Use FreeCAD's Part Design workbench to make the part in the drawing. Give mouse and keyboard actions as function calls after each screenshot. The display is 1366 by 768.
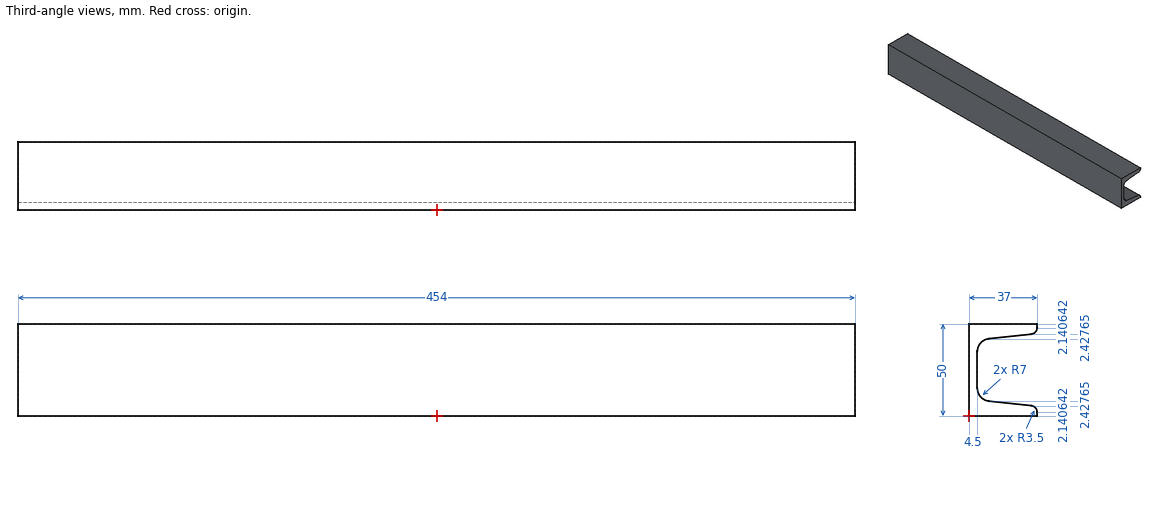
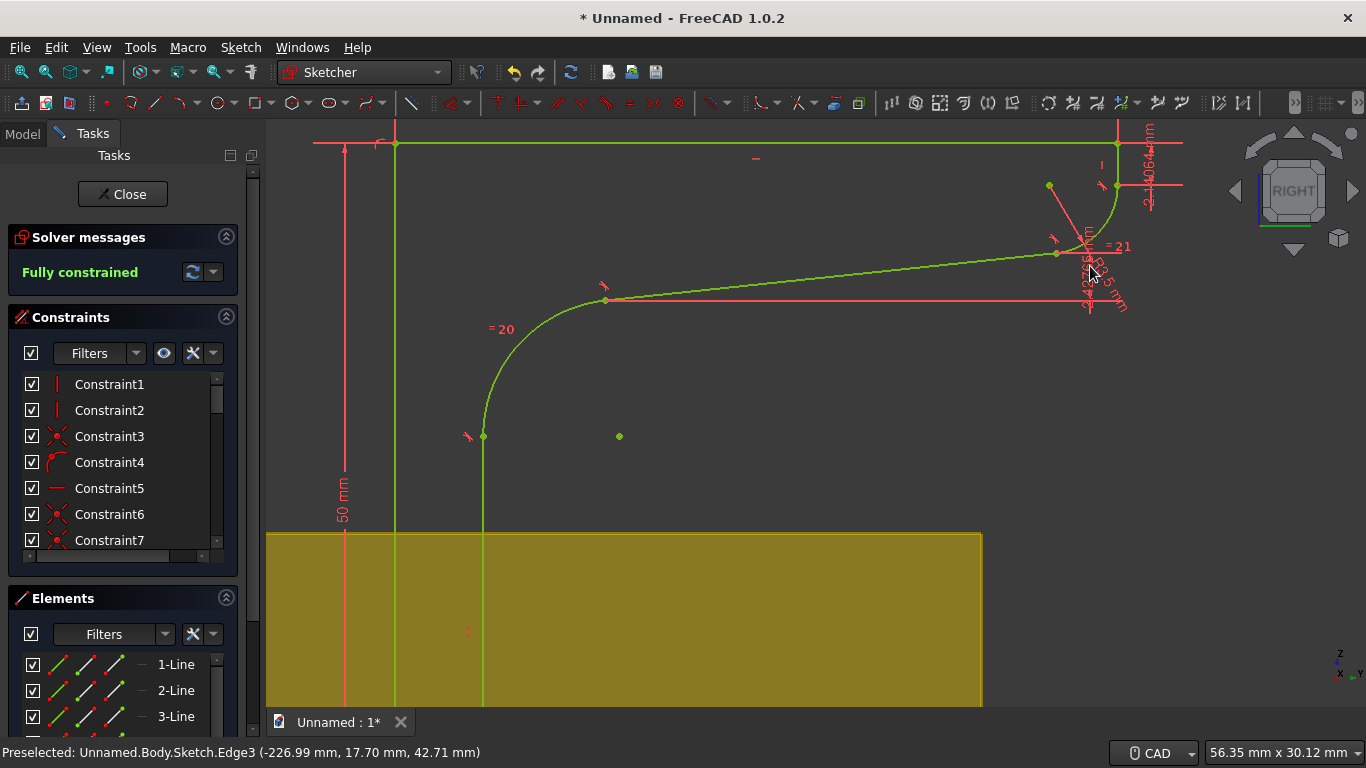
click(123, 194)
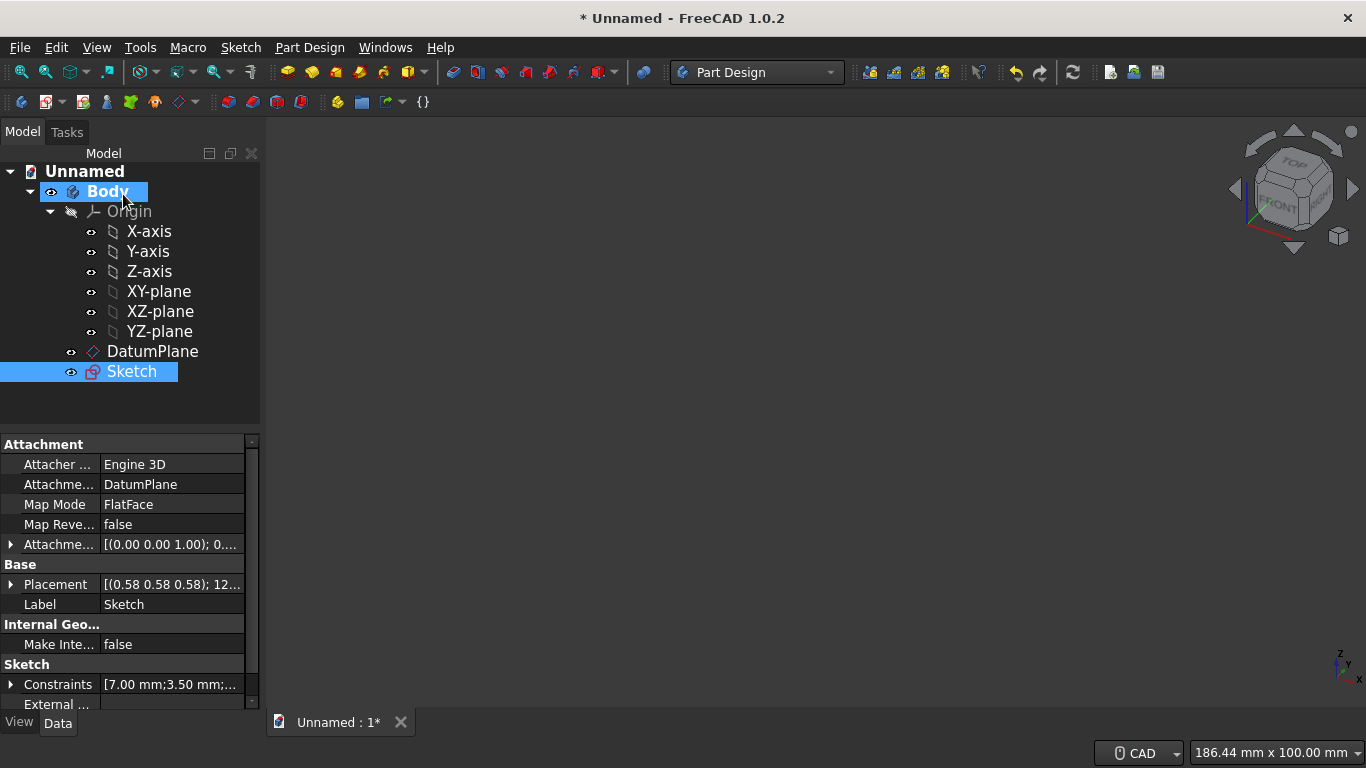
click(288, 72)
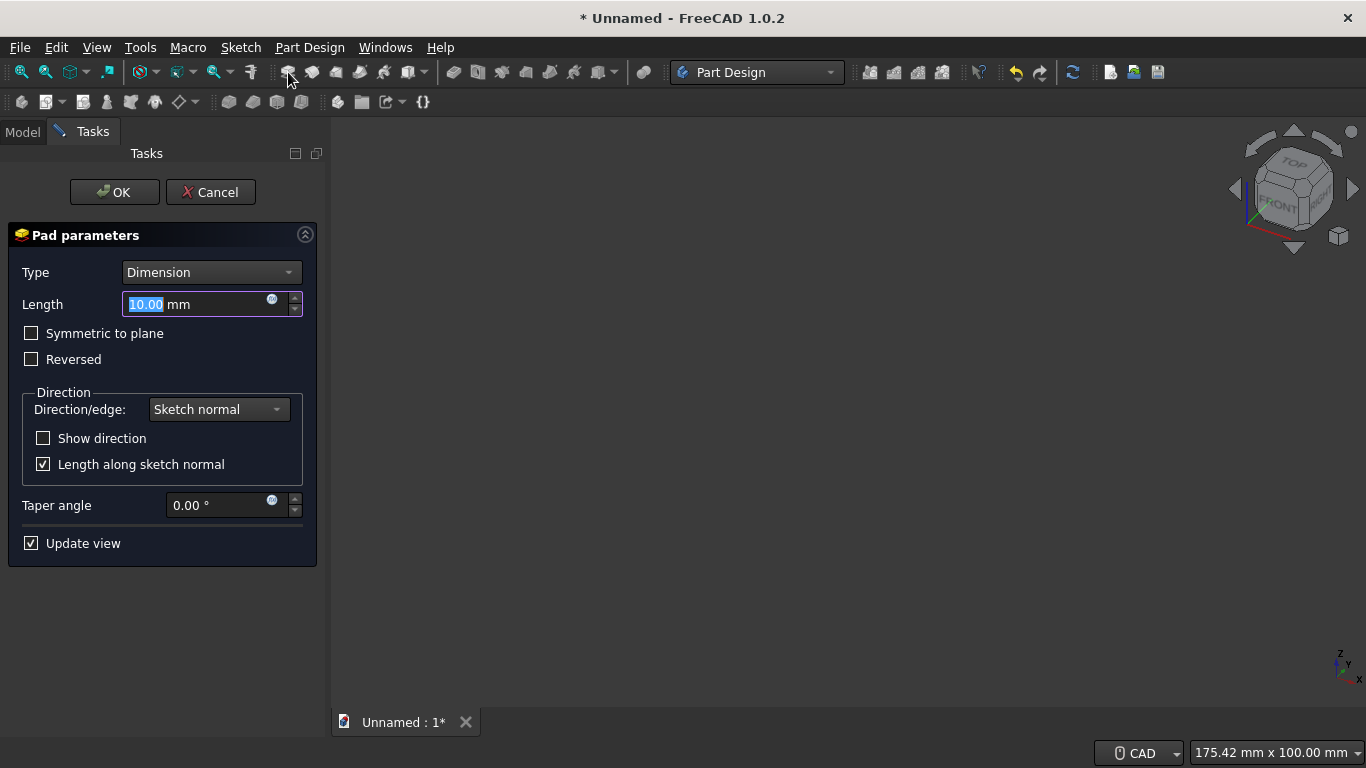
text(454)
key(Tab)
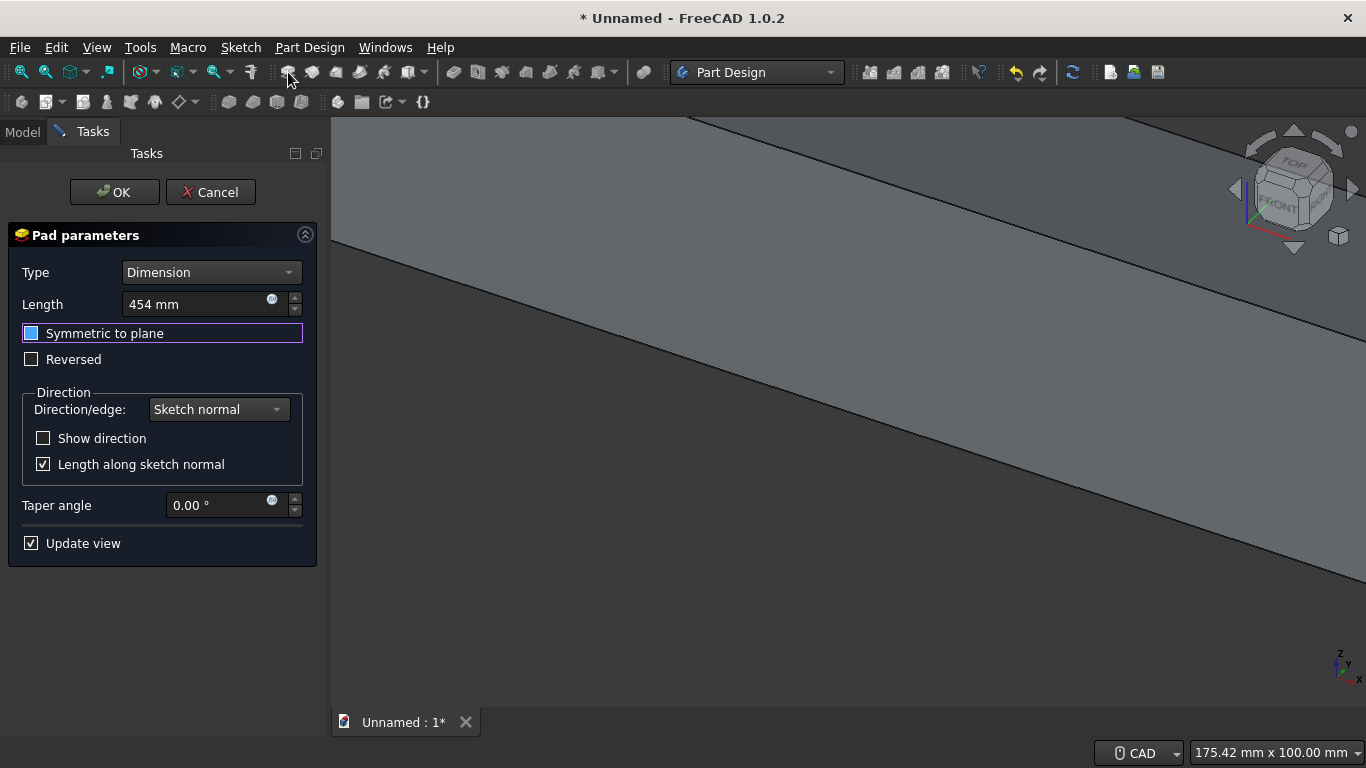
click(115, 192)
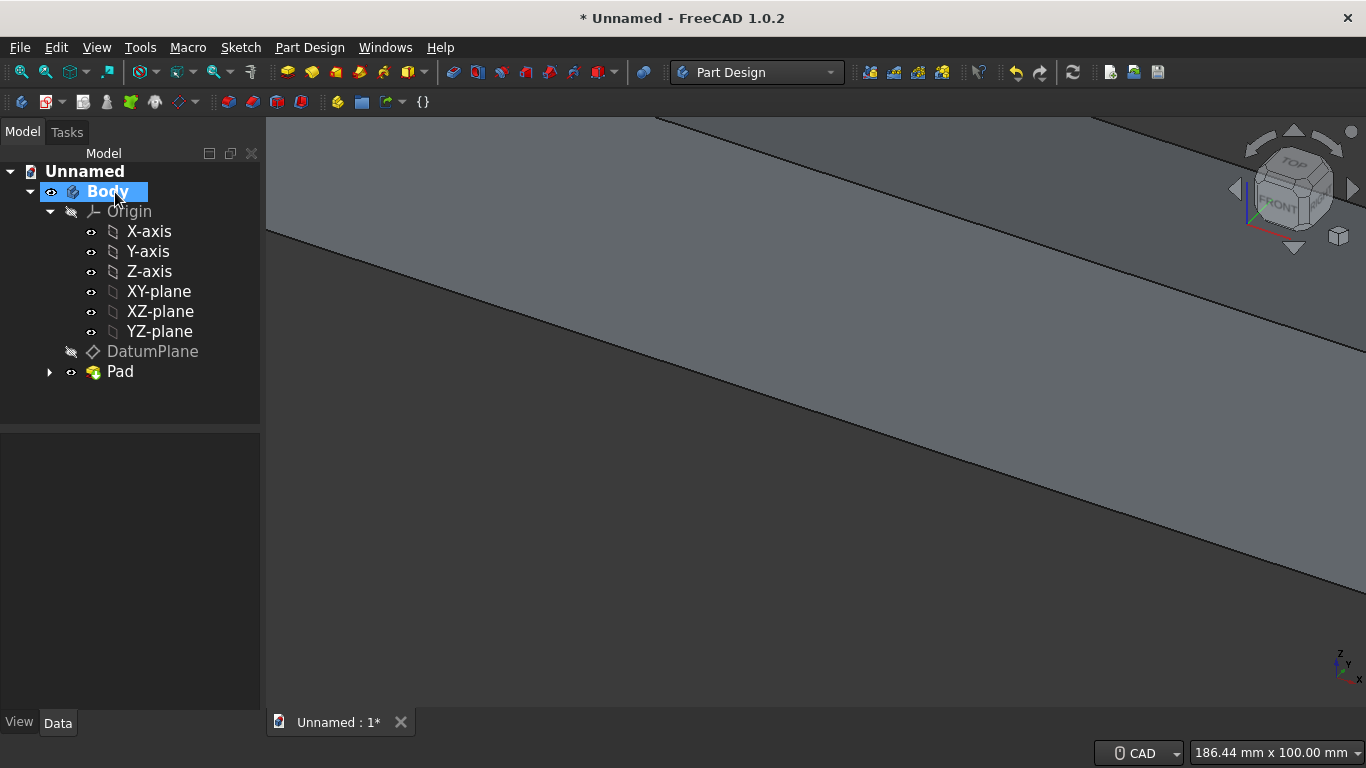
key(0)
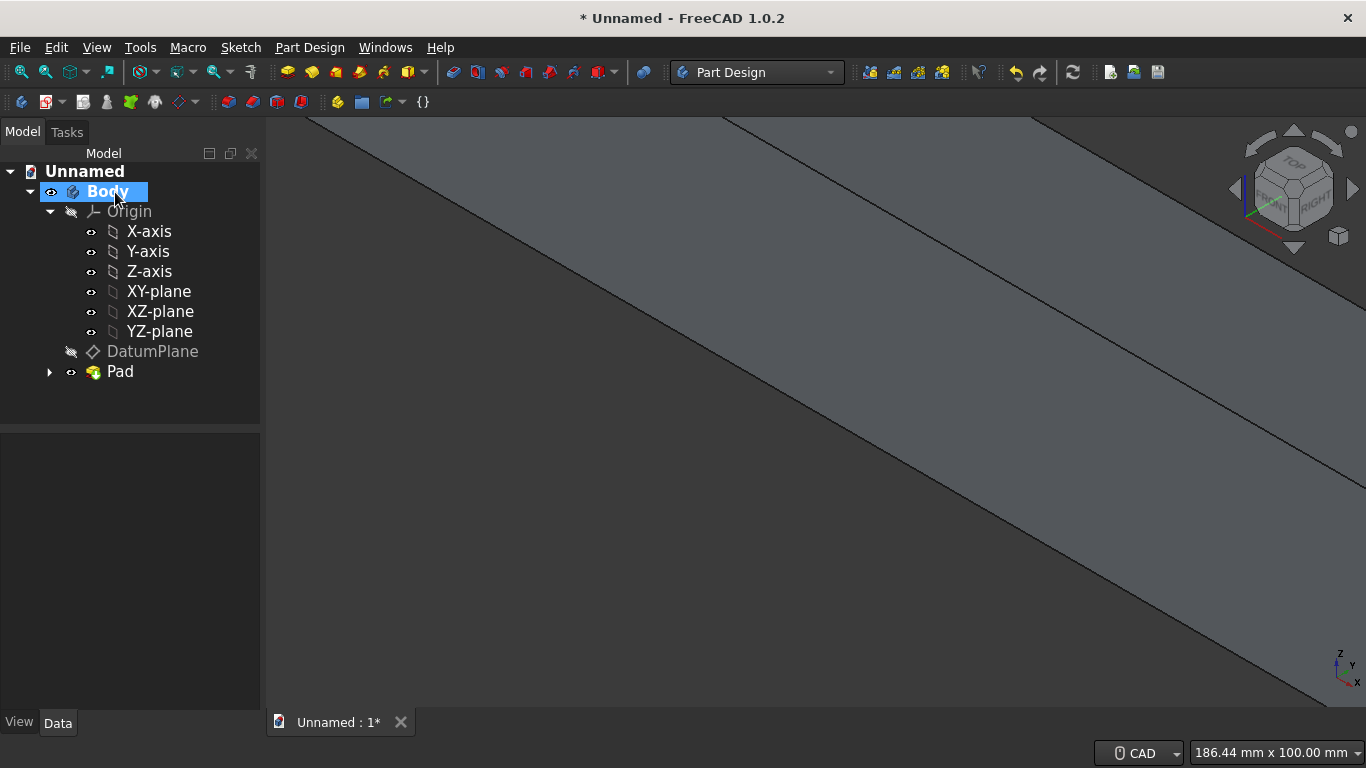
click(22, 72)